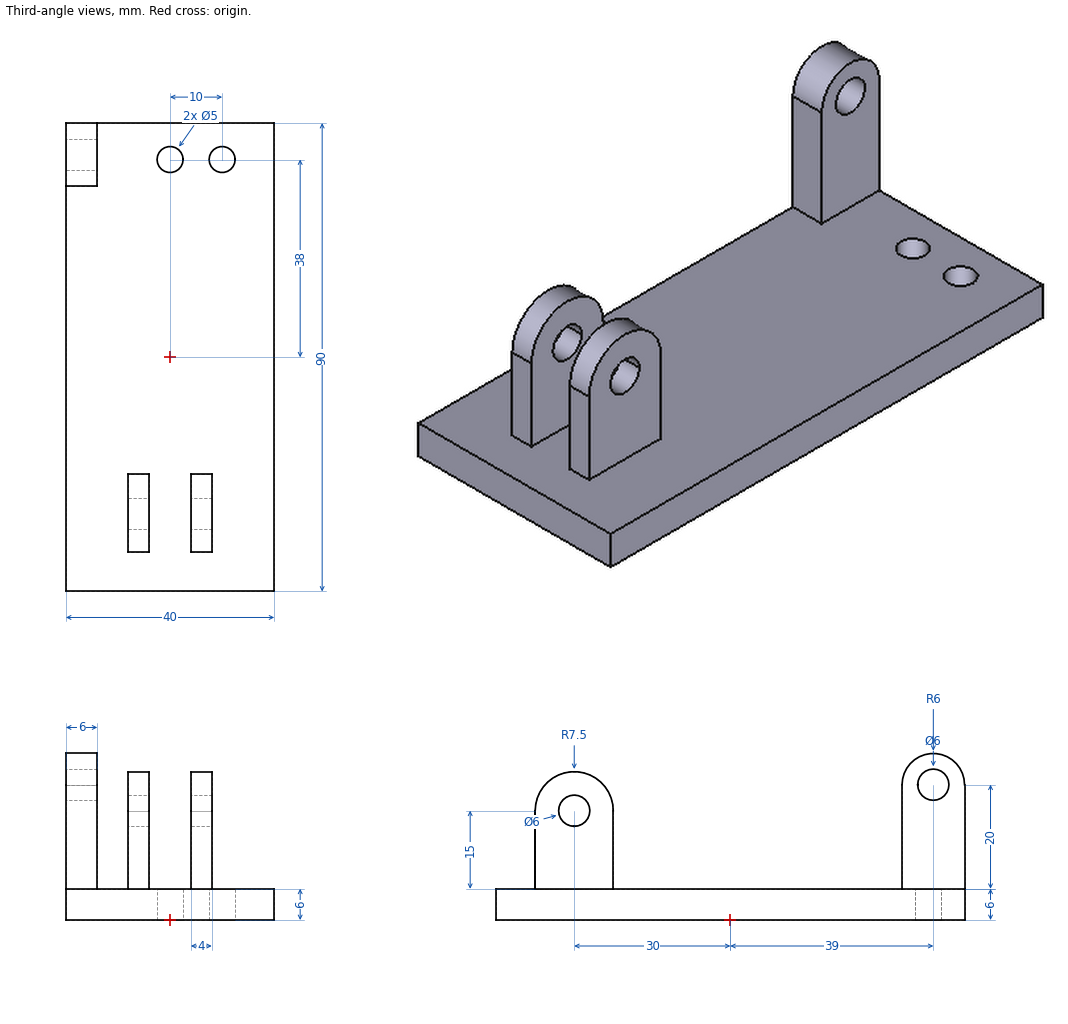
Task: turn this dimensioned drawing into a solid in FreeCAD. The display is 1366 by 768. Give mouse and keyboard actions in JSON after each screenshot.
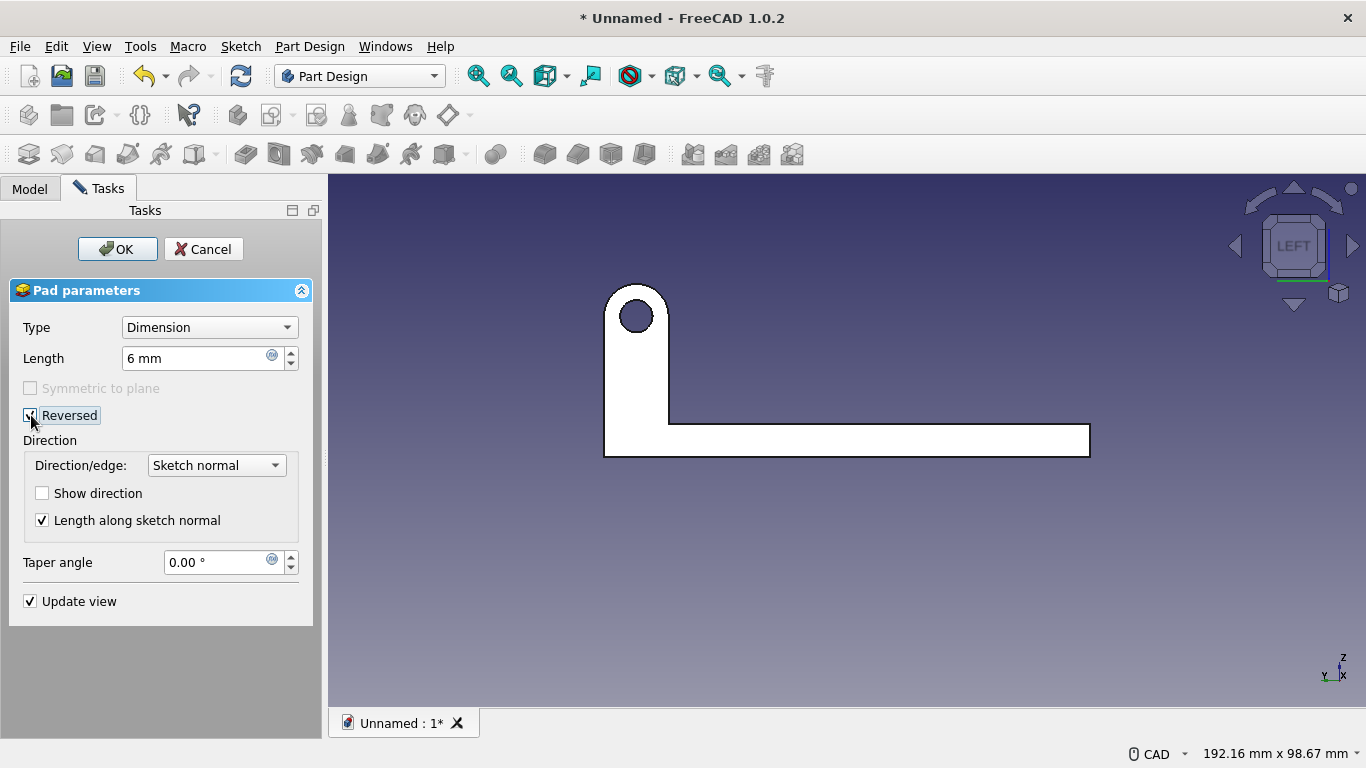
{"action": "left_click", "coordinate": [118, 249]}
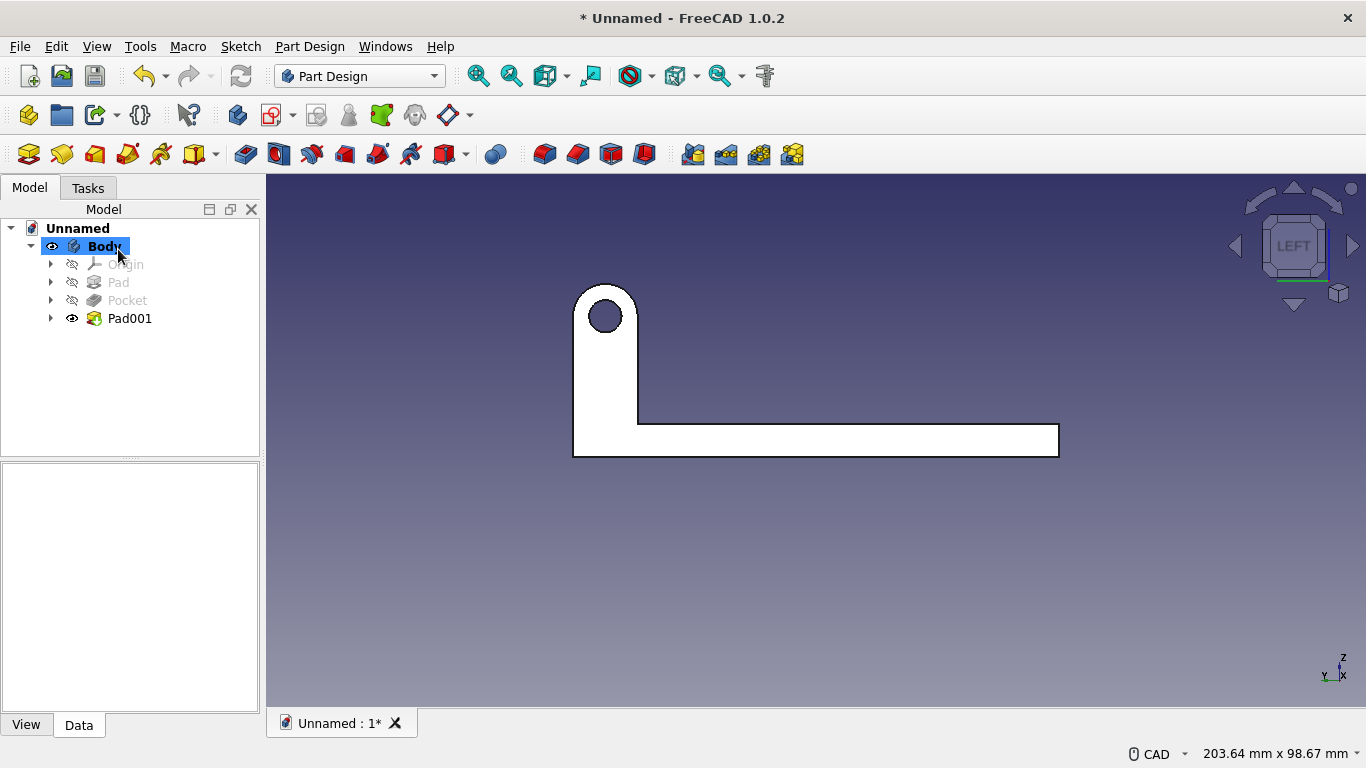
{"action": "left_click", "coordinate": [479, 76]}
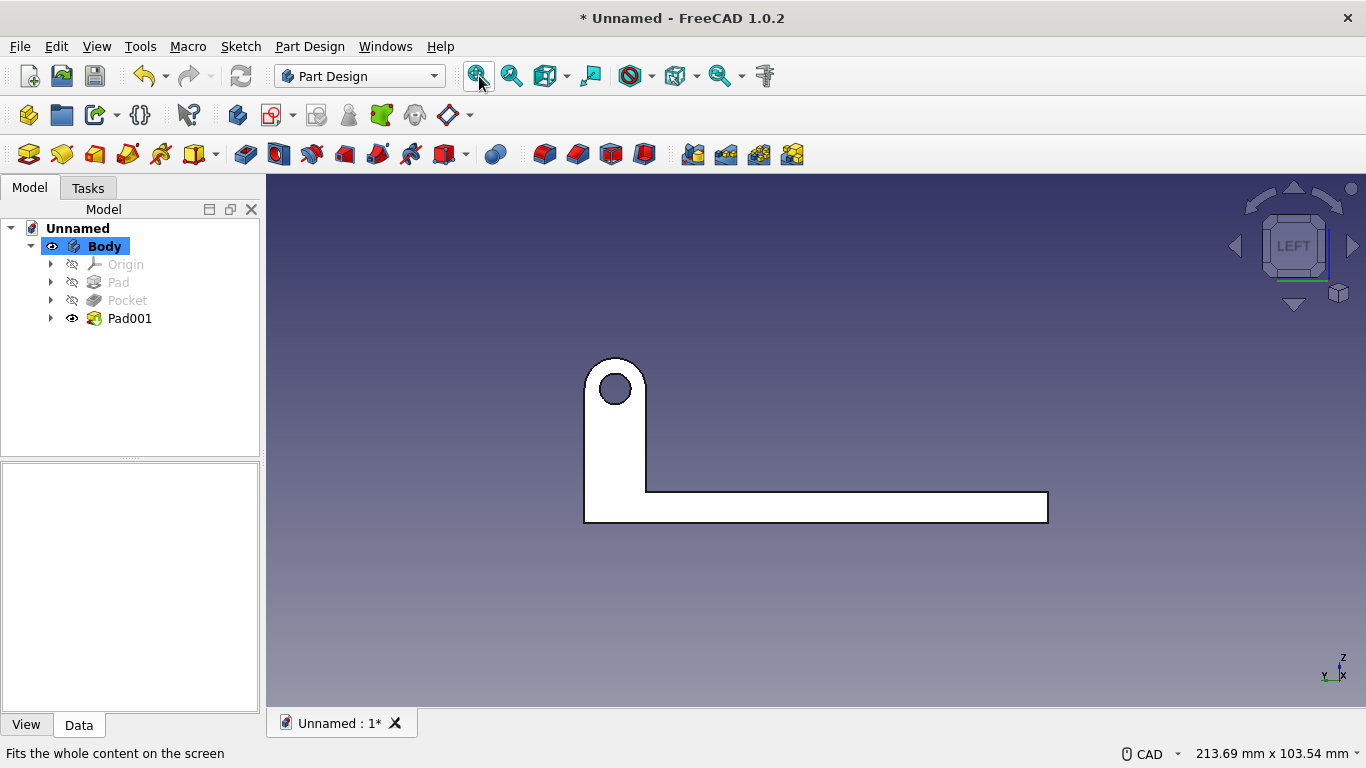
{"action": "left_click", "coordinate": [51, 264]}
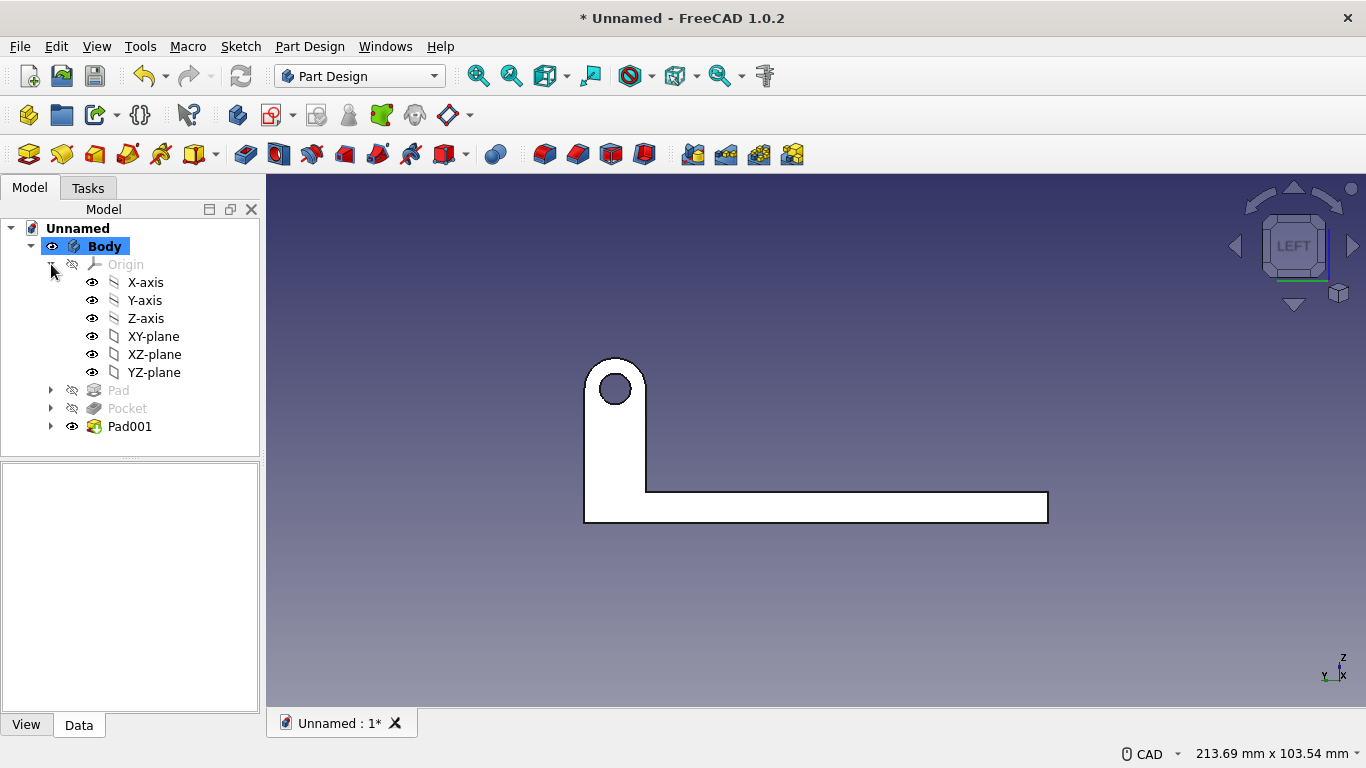
{"action": "left_click", "coordinate": [137, 372]}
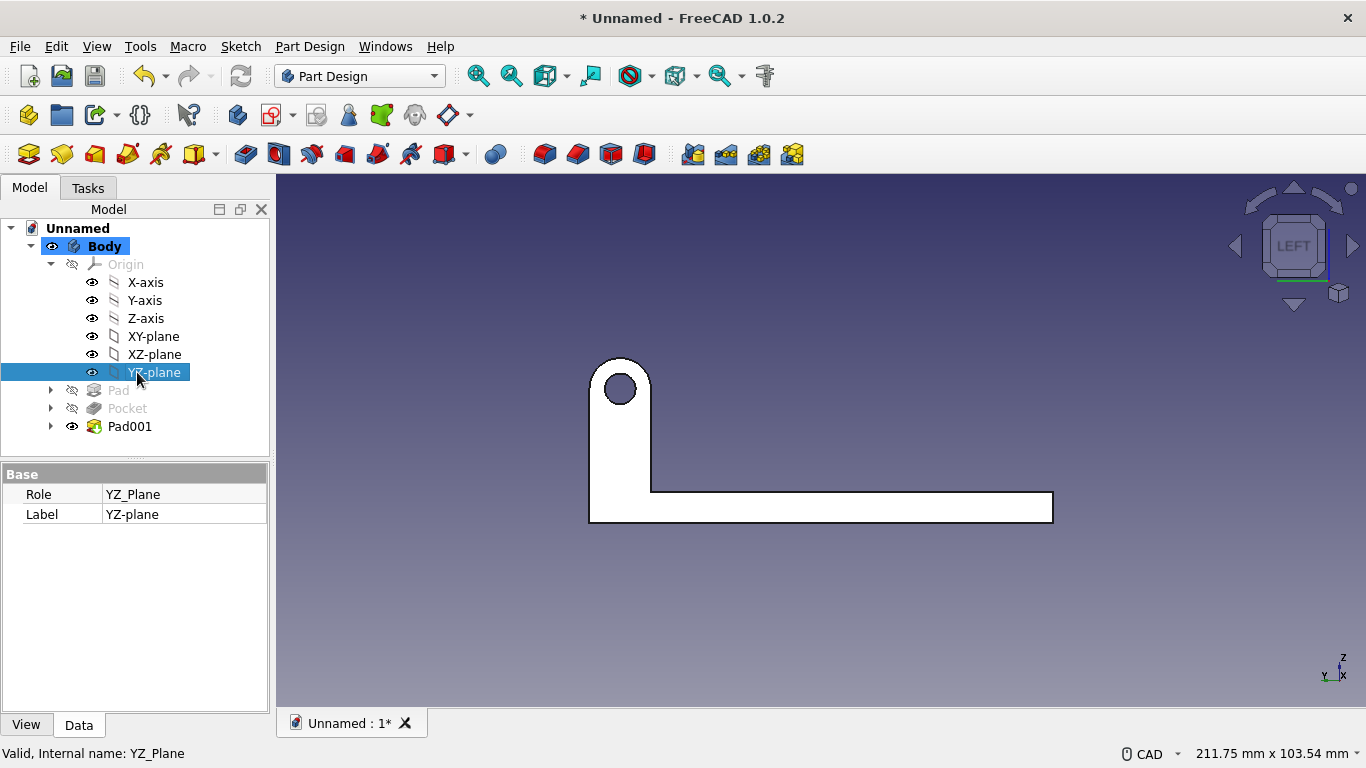
{"action": "left_click", "coordinate": [448, 116]}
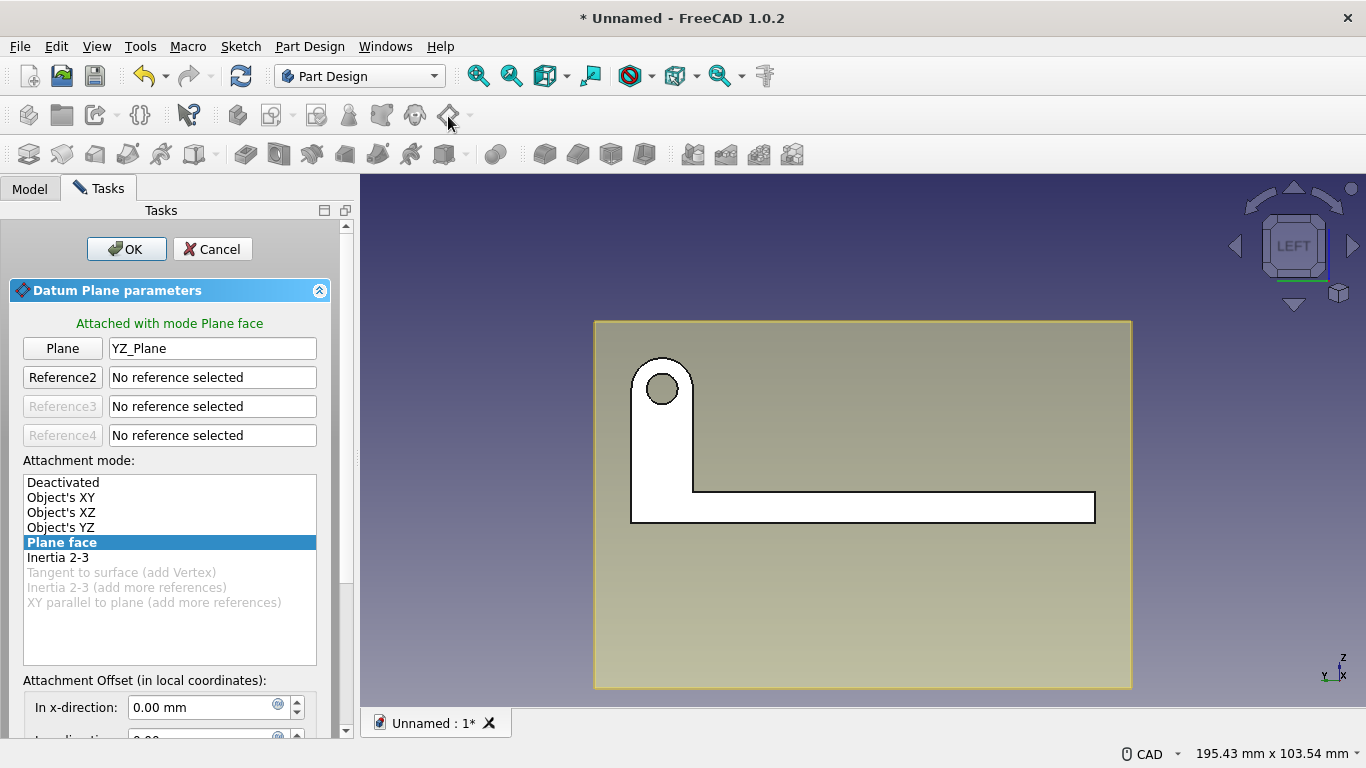
{"action": "scroll", "coordinate": [346, 479], "scroll_direction": "down", "scroll_amount": 2}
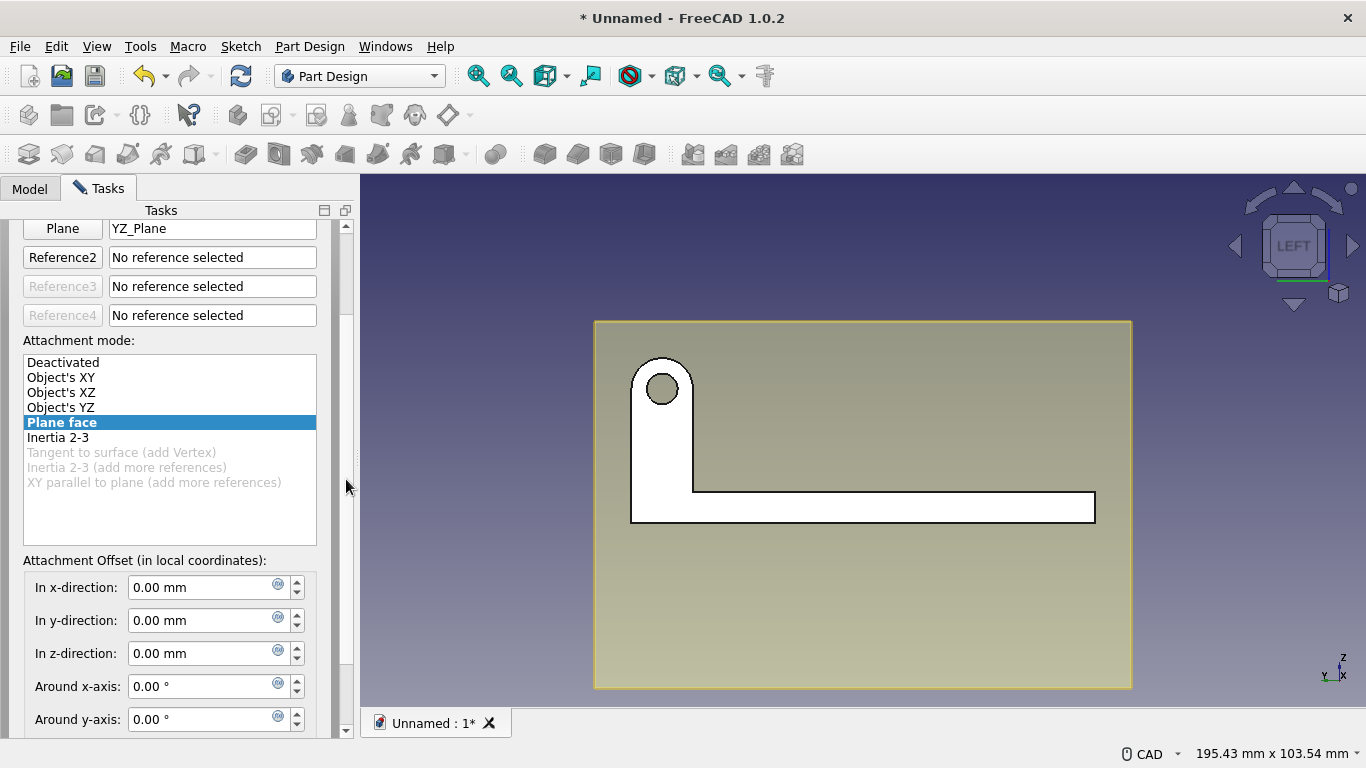
{"action": "triple_click", "coordinate": [210, 654]}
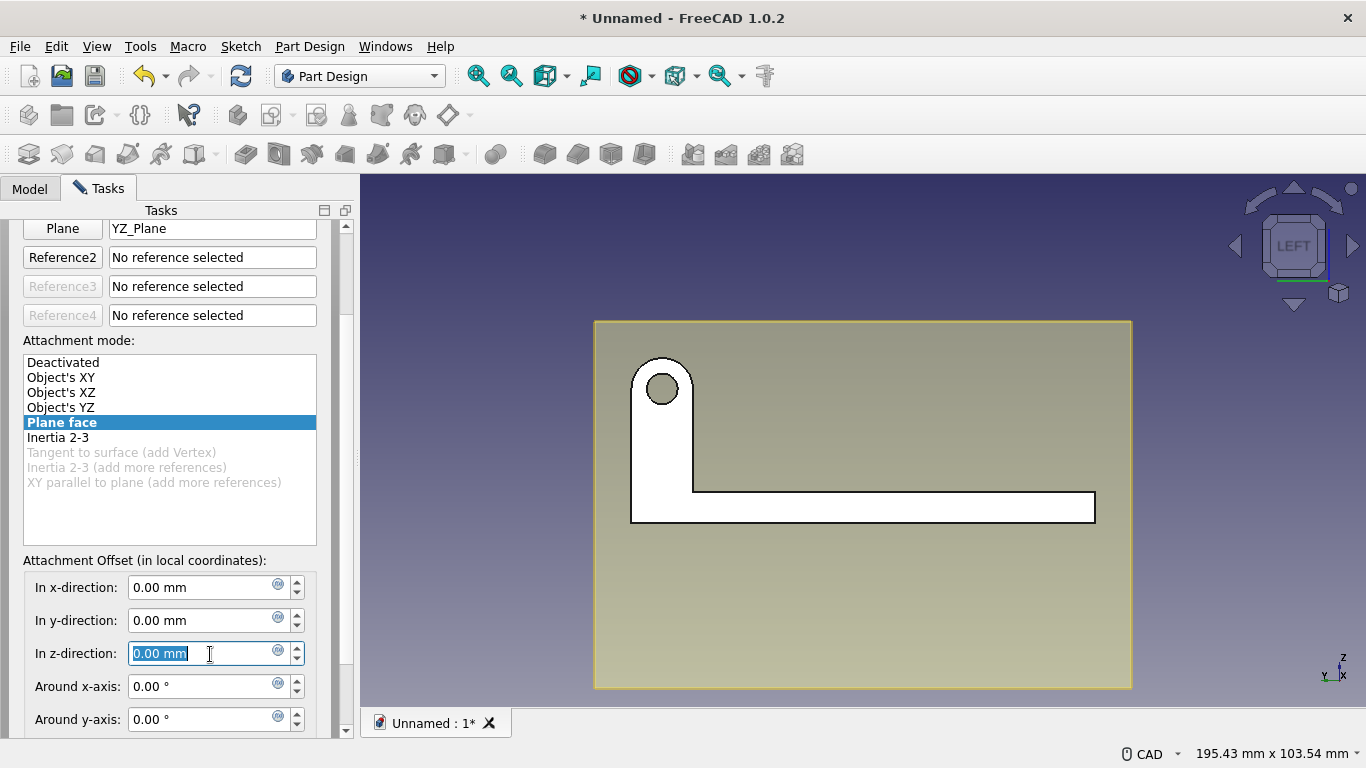
{"action": "type", "text": "4"}
{"action": "key", "text": "Tab"}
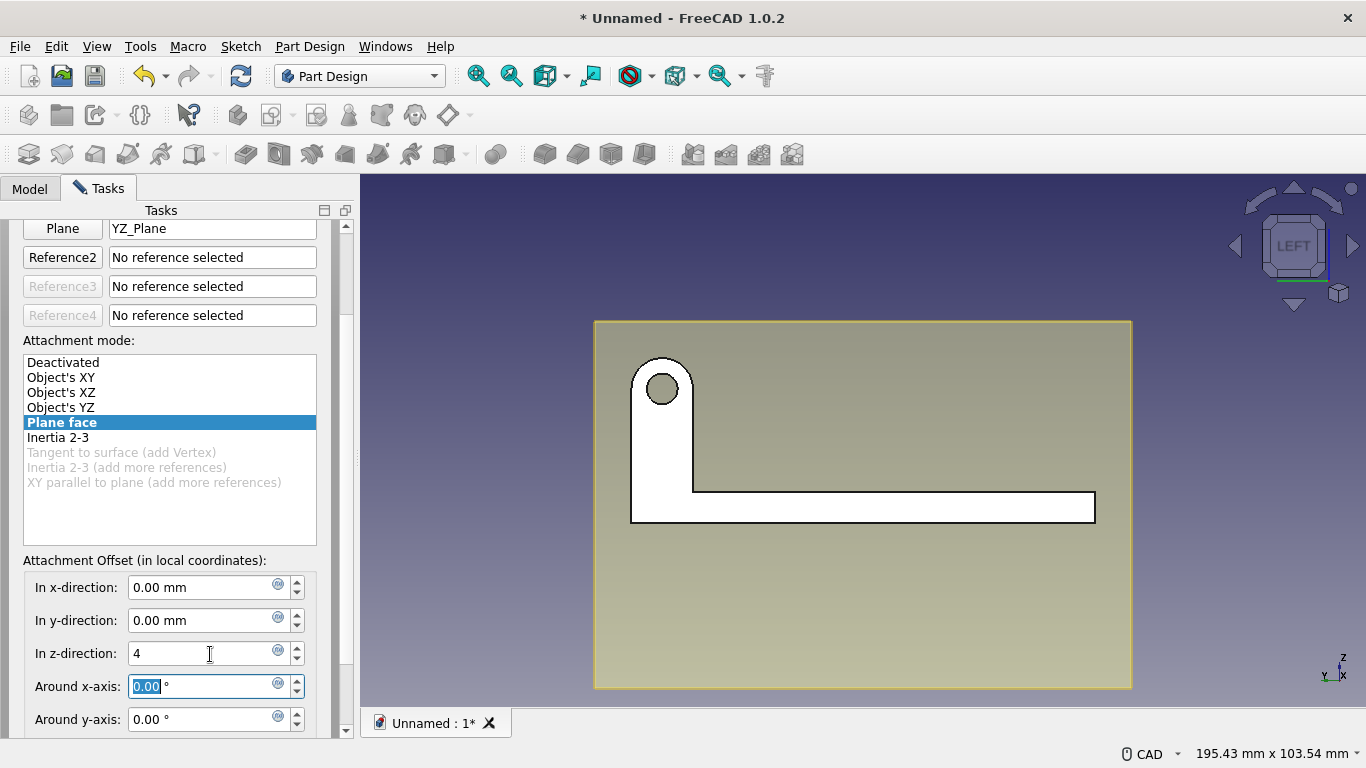
{"action": "scroll", "coordinate": [346, 479], "scroll_direction": "up", "scroll_amount": 3}